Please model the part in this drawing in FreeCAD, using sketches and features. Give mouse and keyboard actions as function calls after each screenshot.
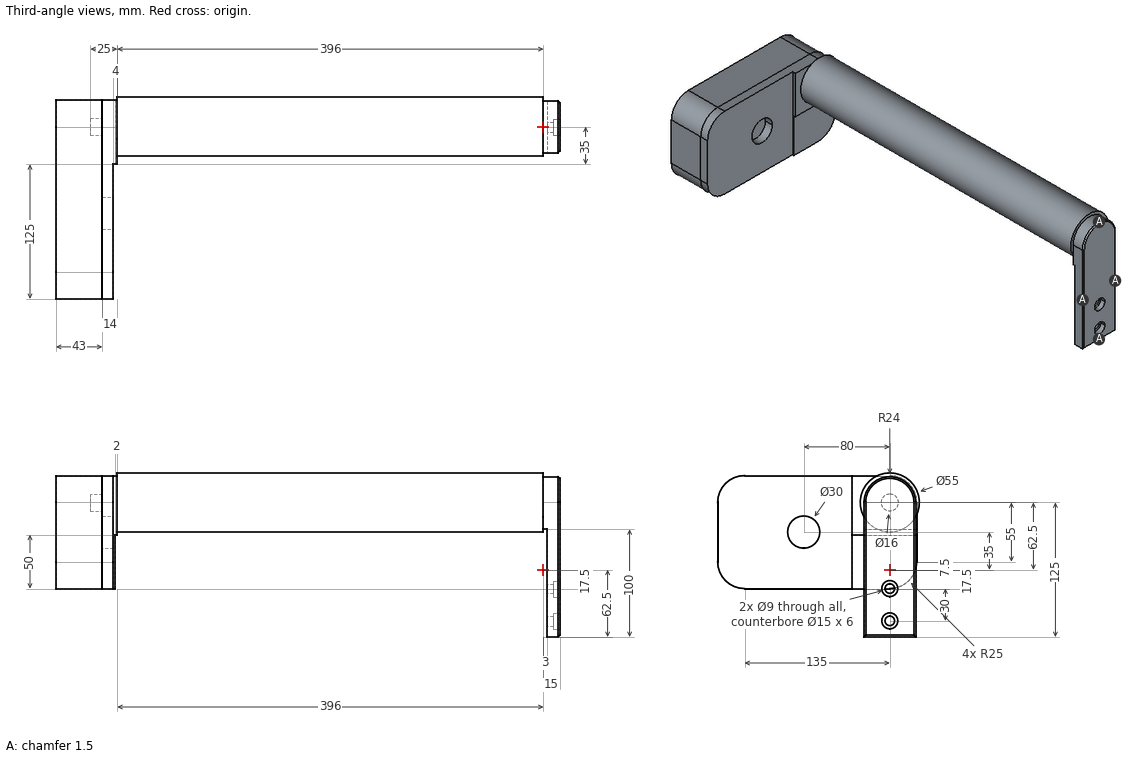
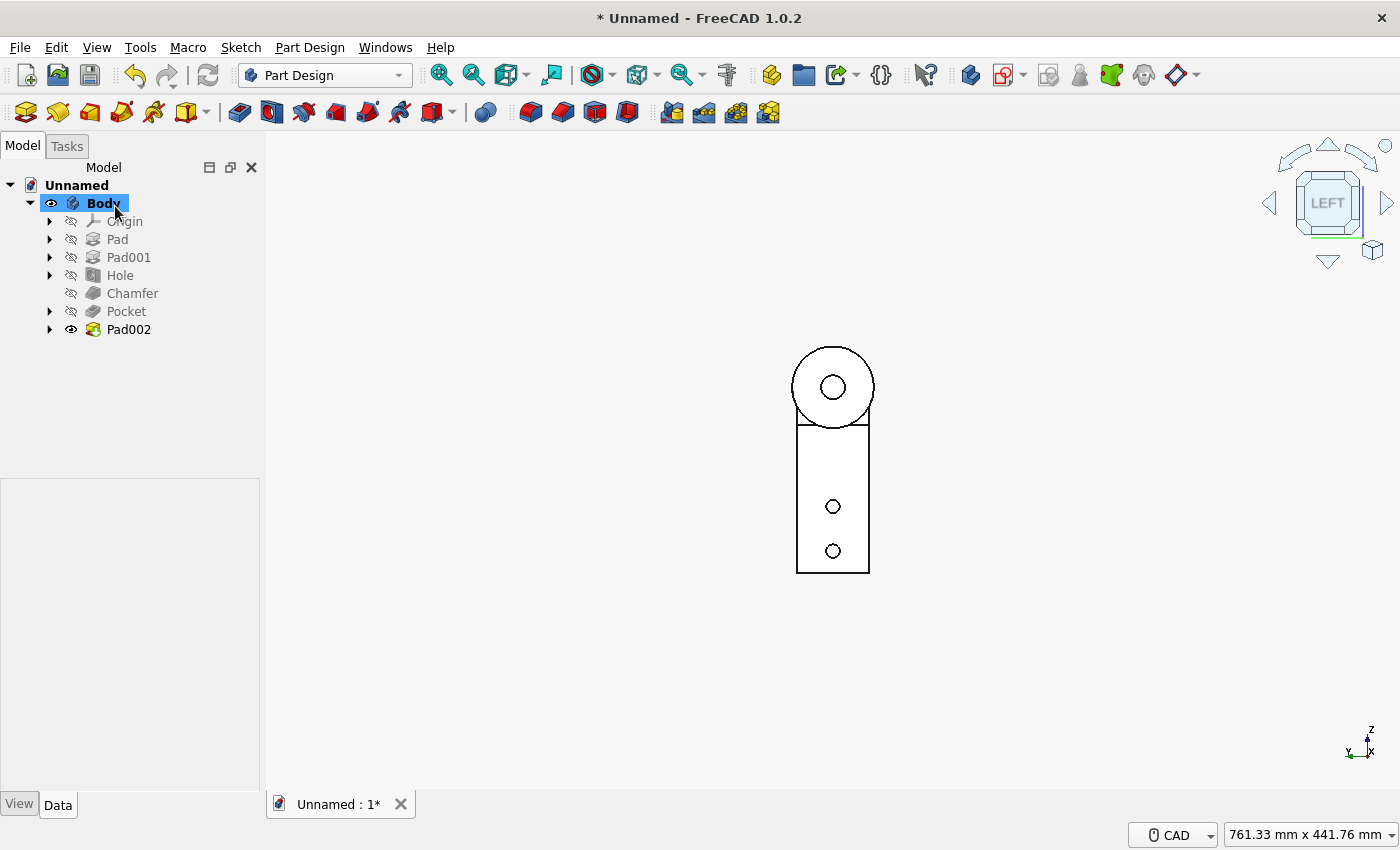
key(v)
key(f)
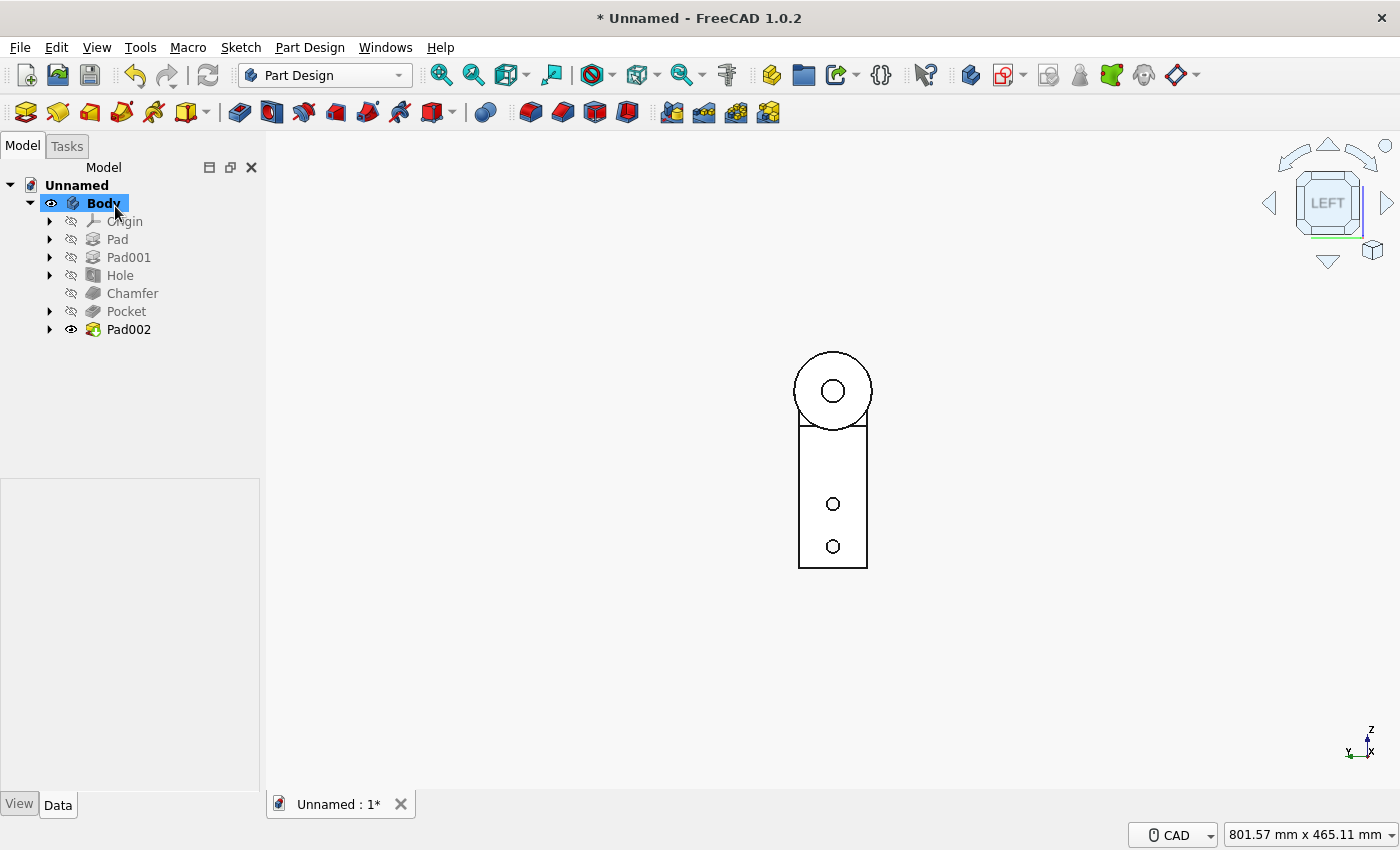
click(822, 368)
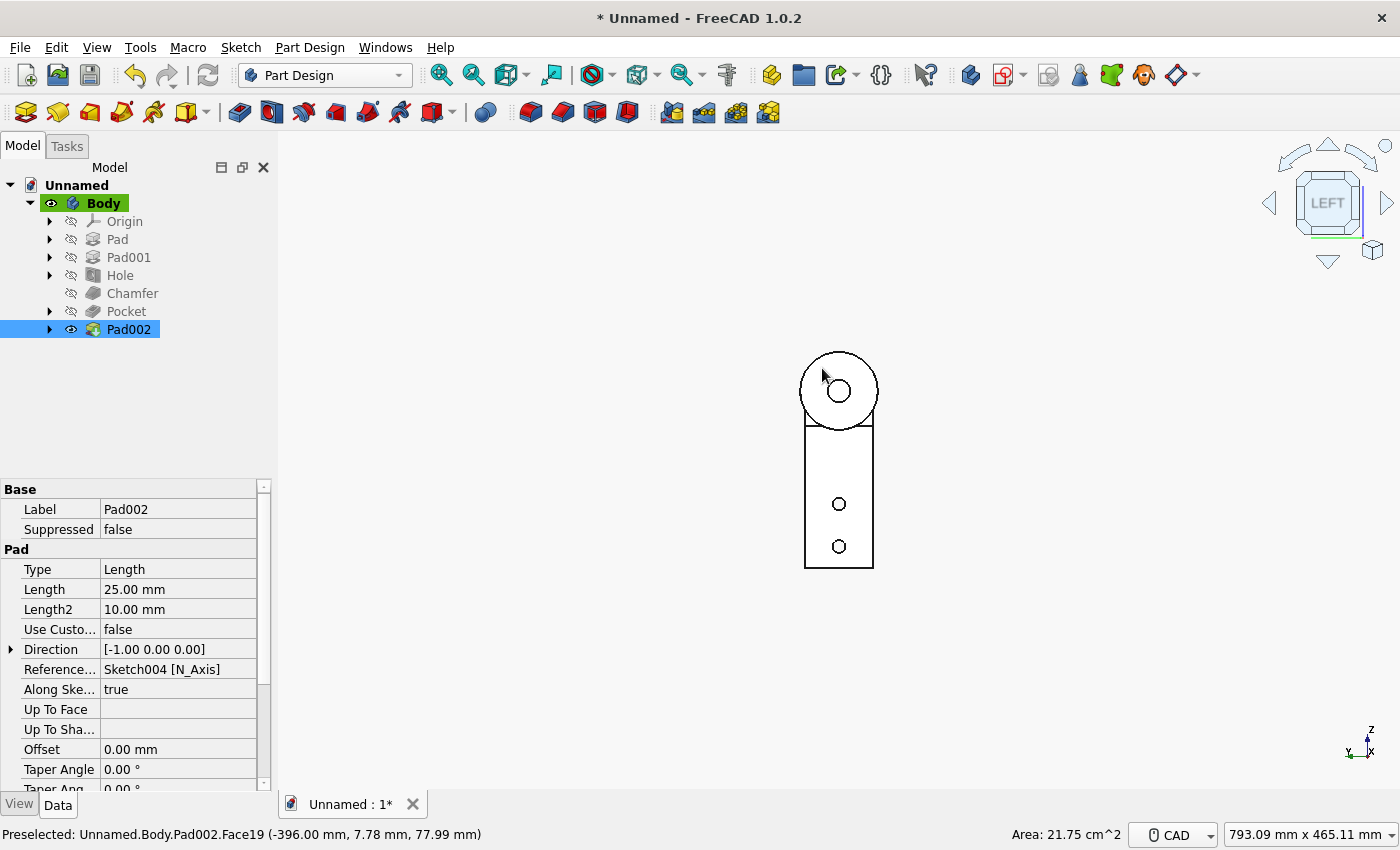
click(1004, 76)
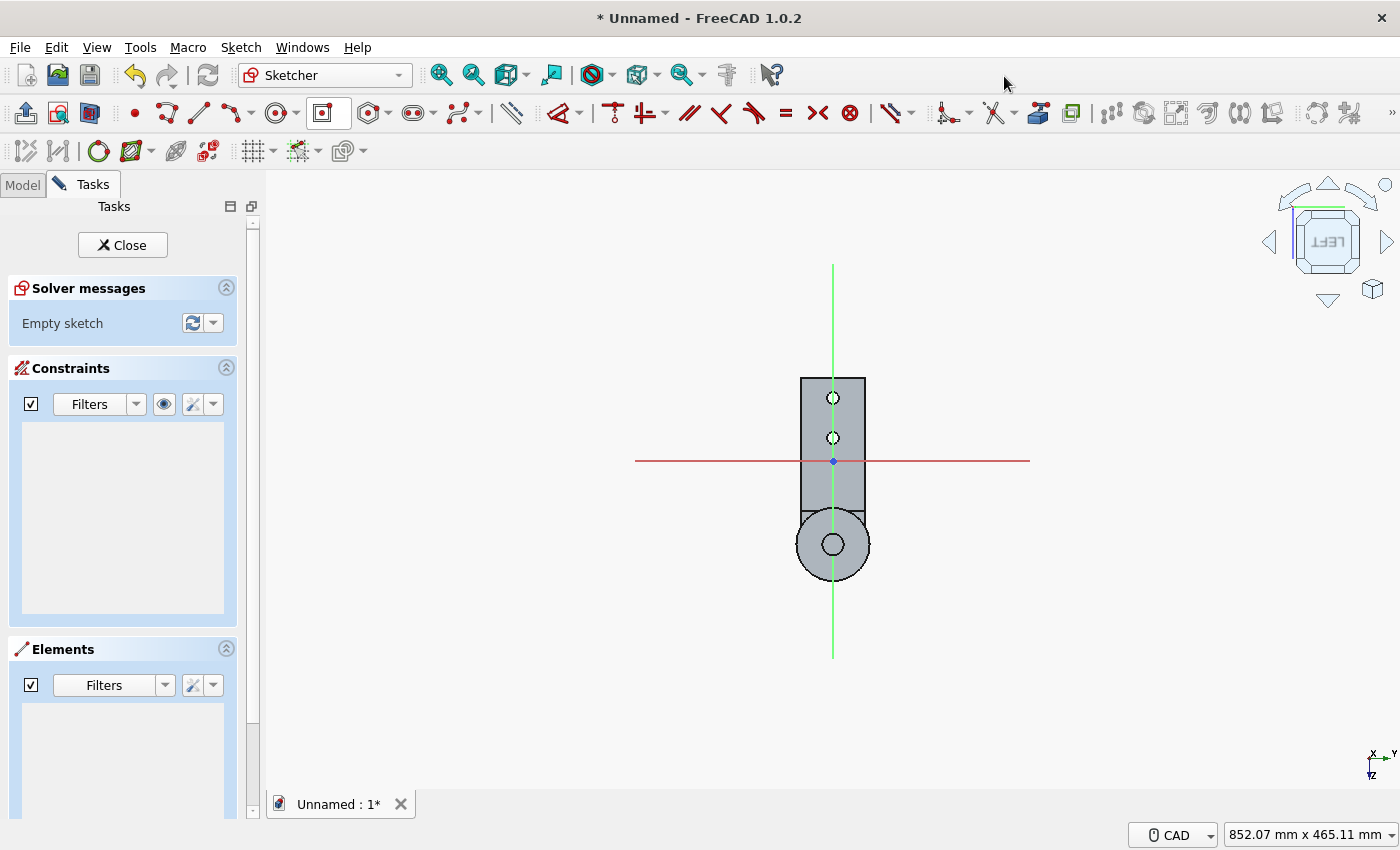
key(q)
key(s)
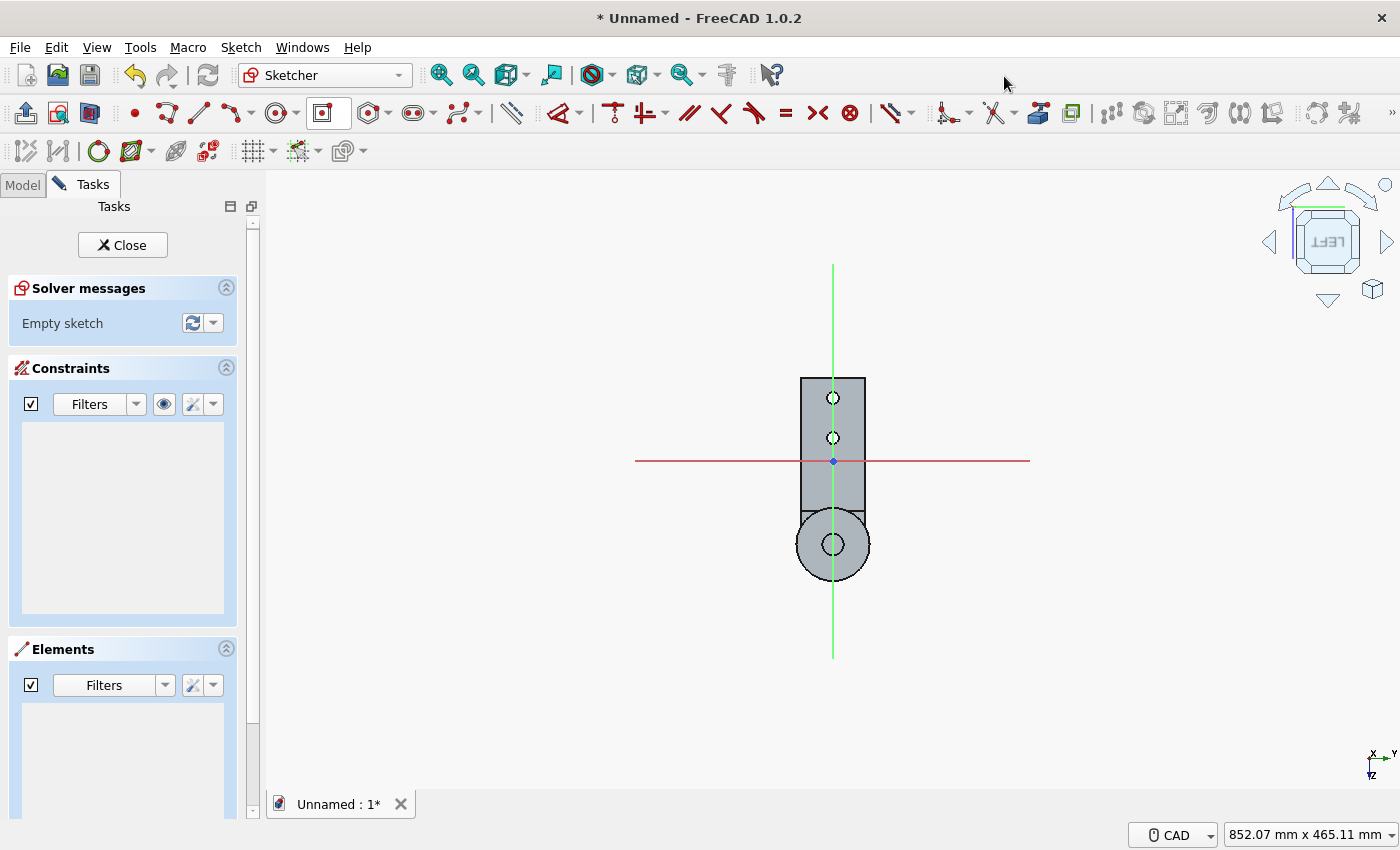
scroll(731, 524, up, 5)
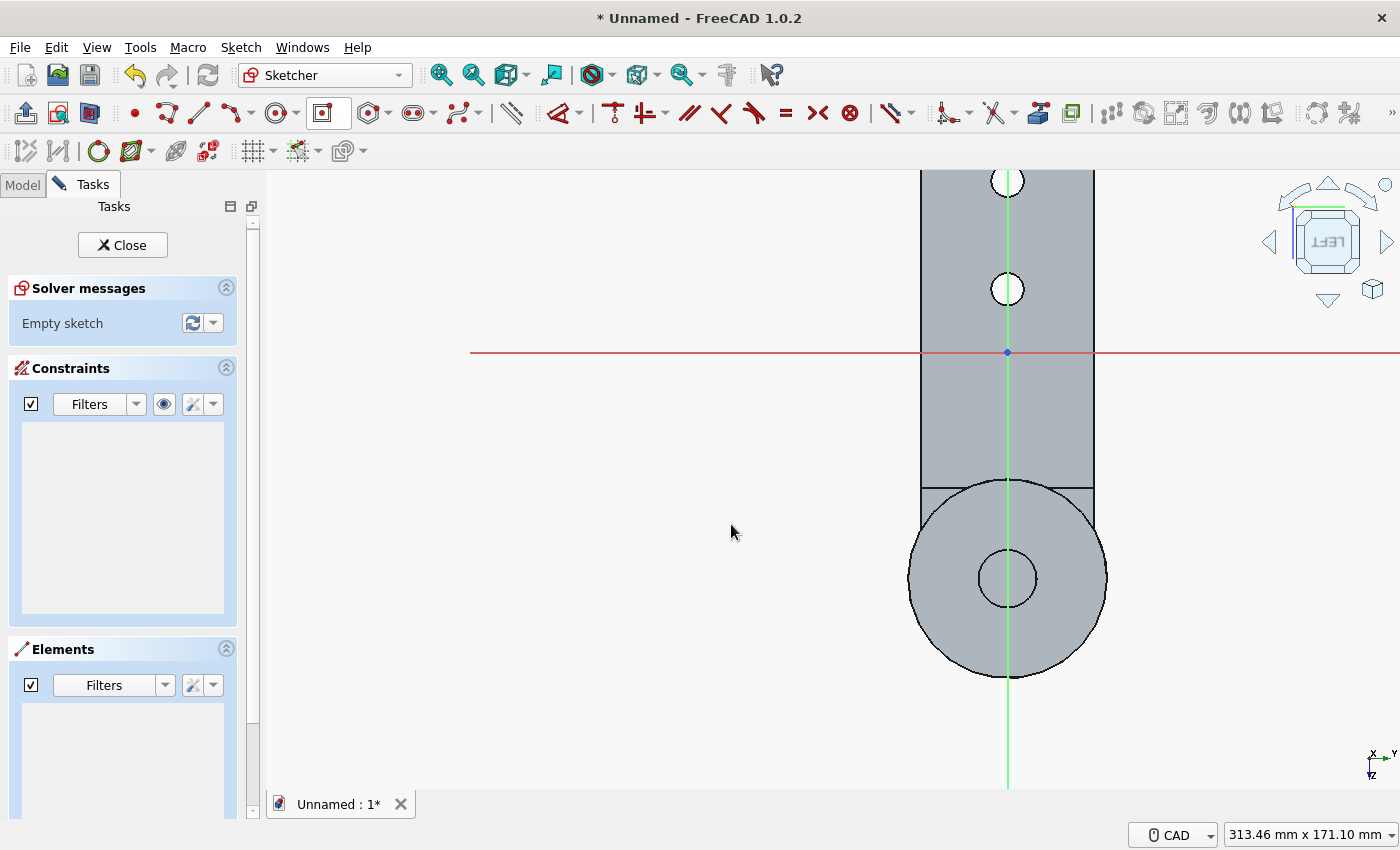
key(g)
key(l)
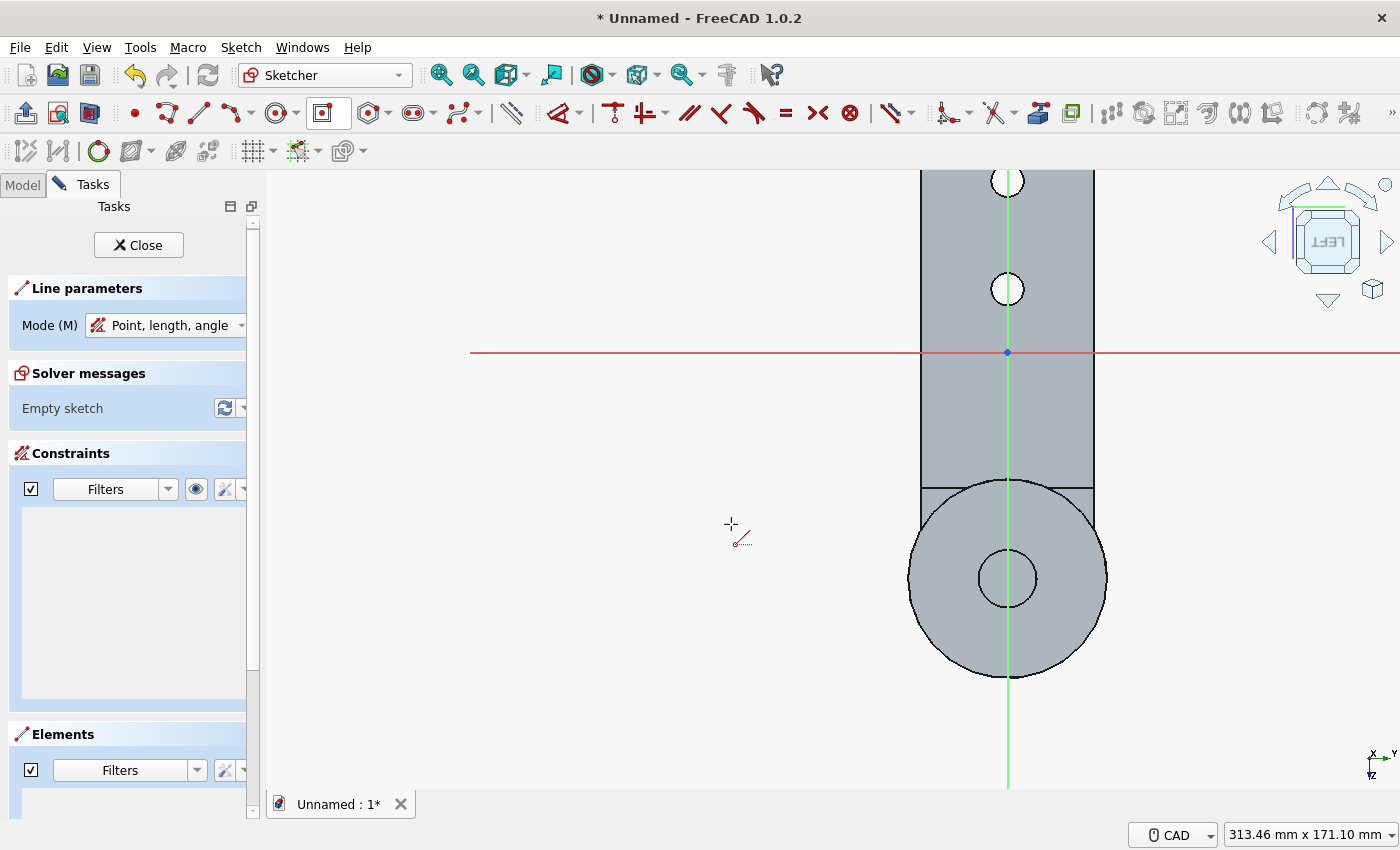
click(1098, 579)
click(1098, 380)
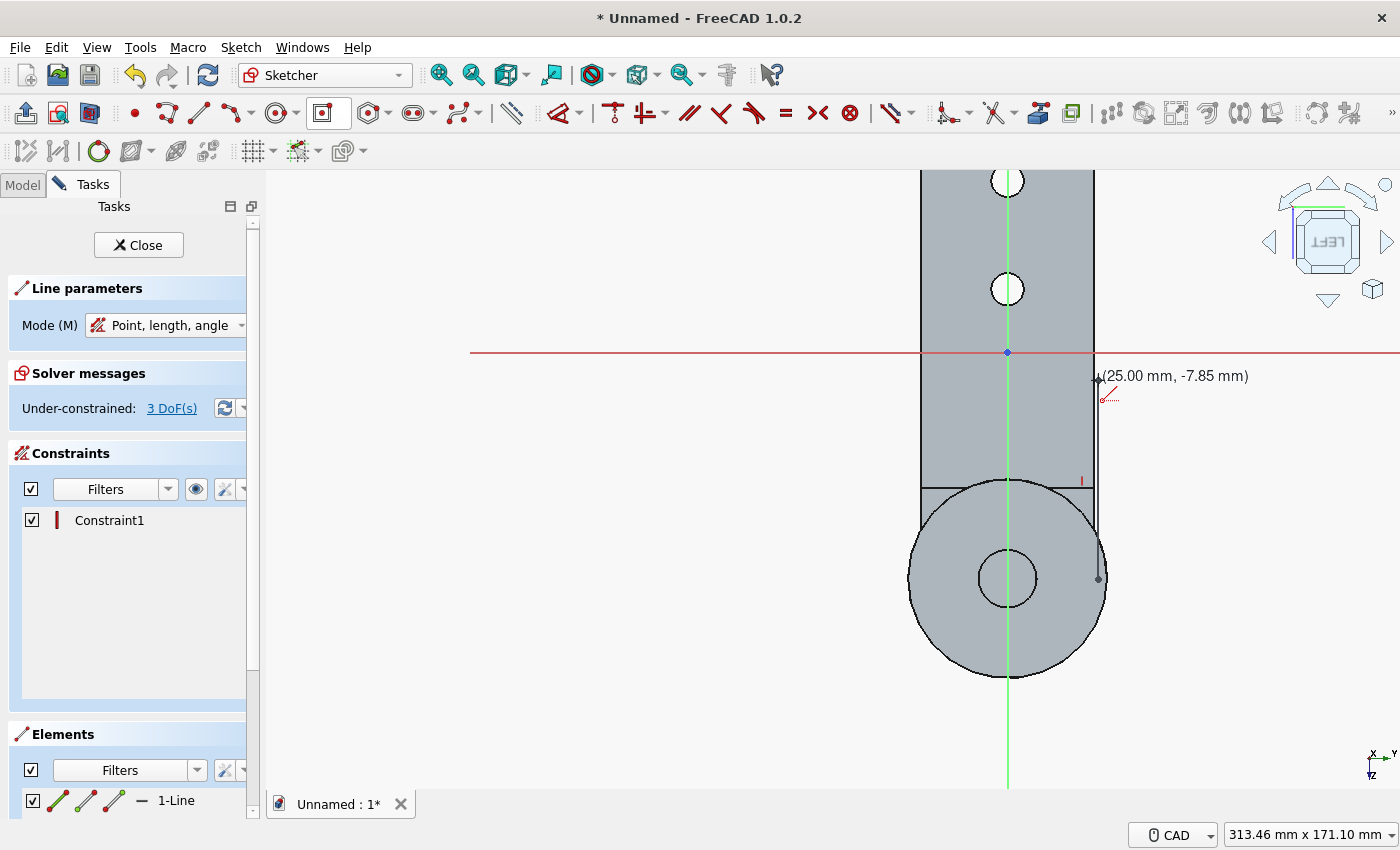
click(1008, 289)
click(519, 289)